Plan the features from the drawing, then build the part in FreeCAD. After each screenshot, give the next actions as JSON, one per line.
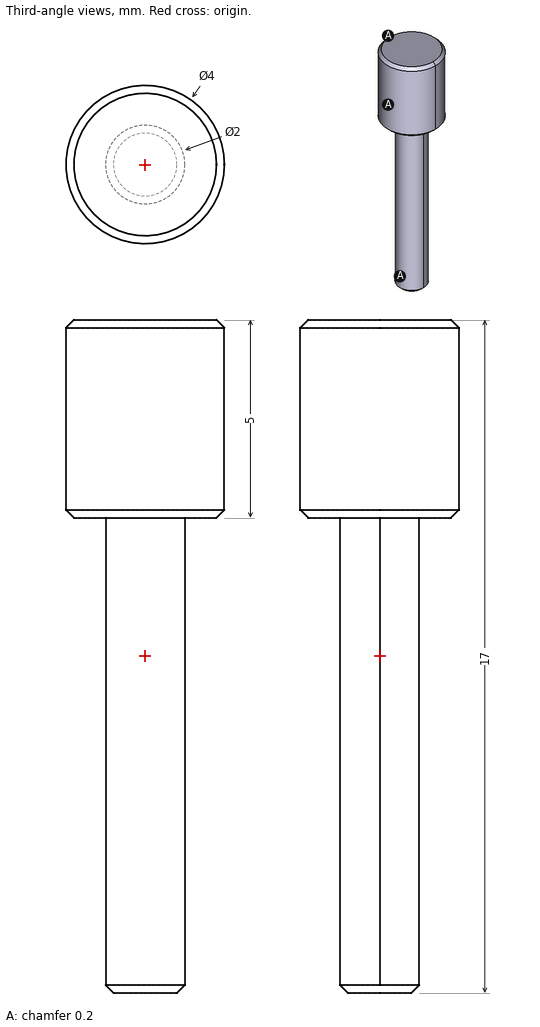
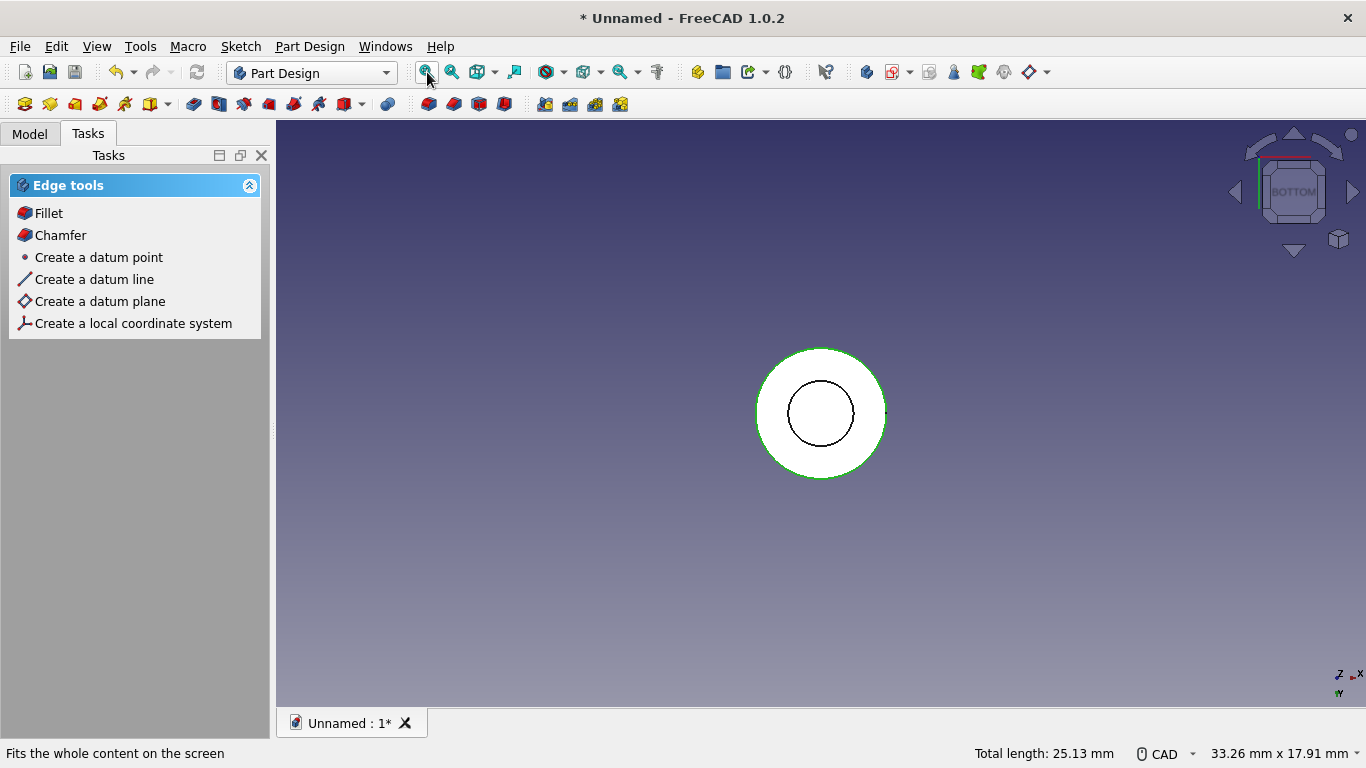
{"action": "left_click", "coordinate": [788, 412], "text": "ctrl"}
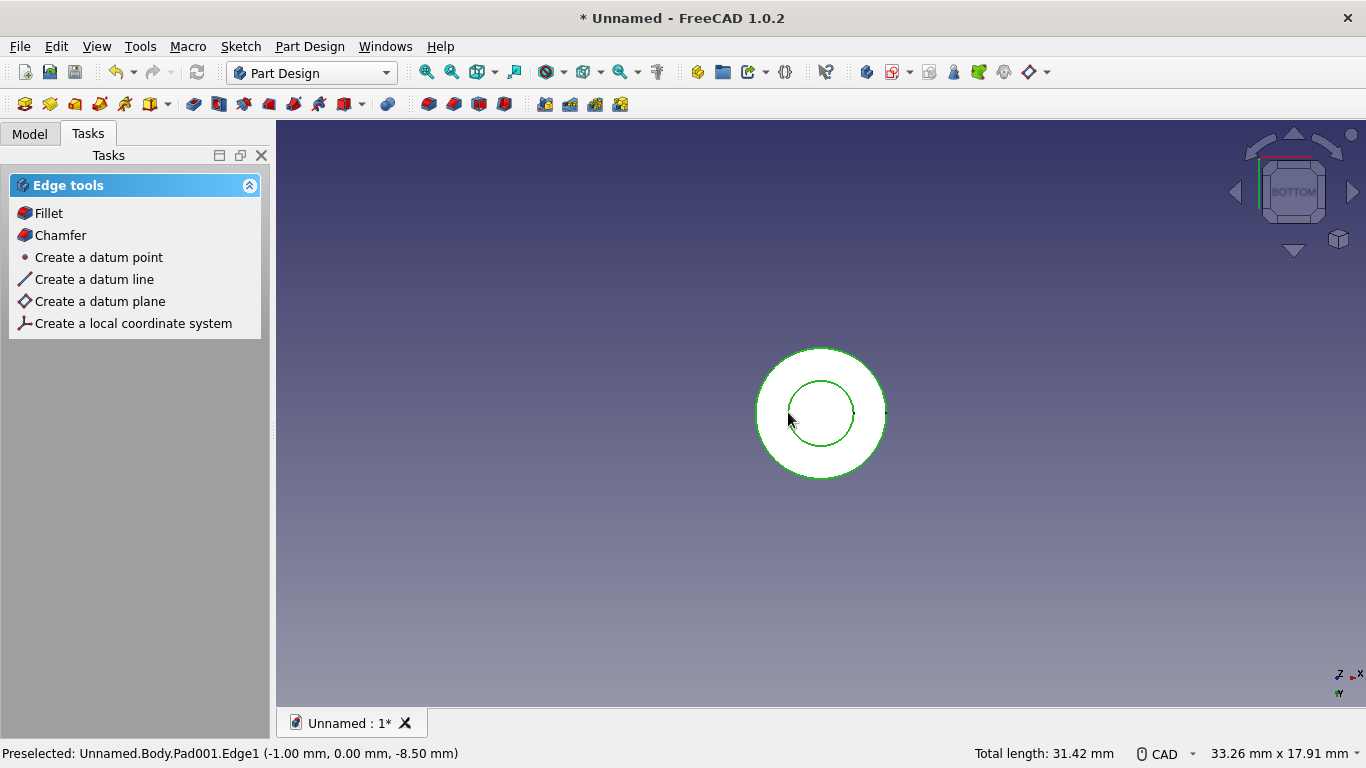
{"action": "left_click", "coordinate": [454, 104]}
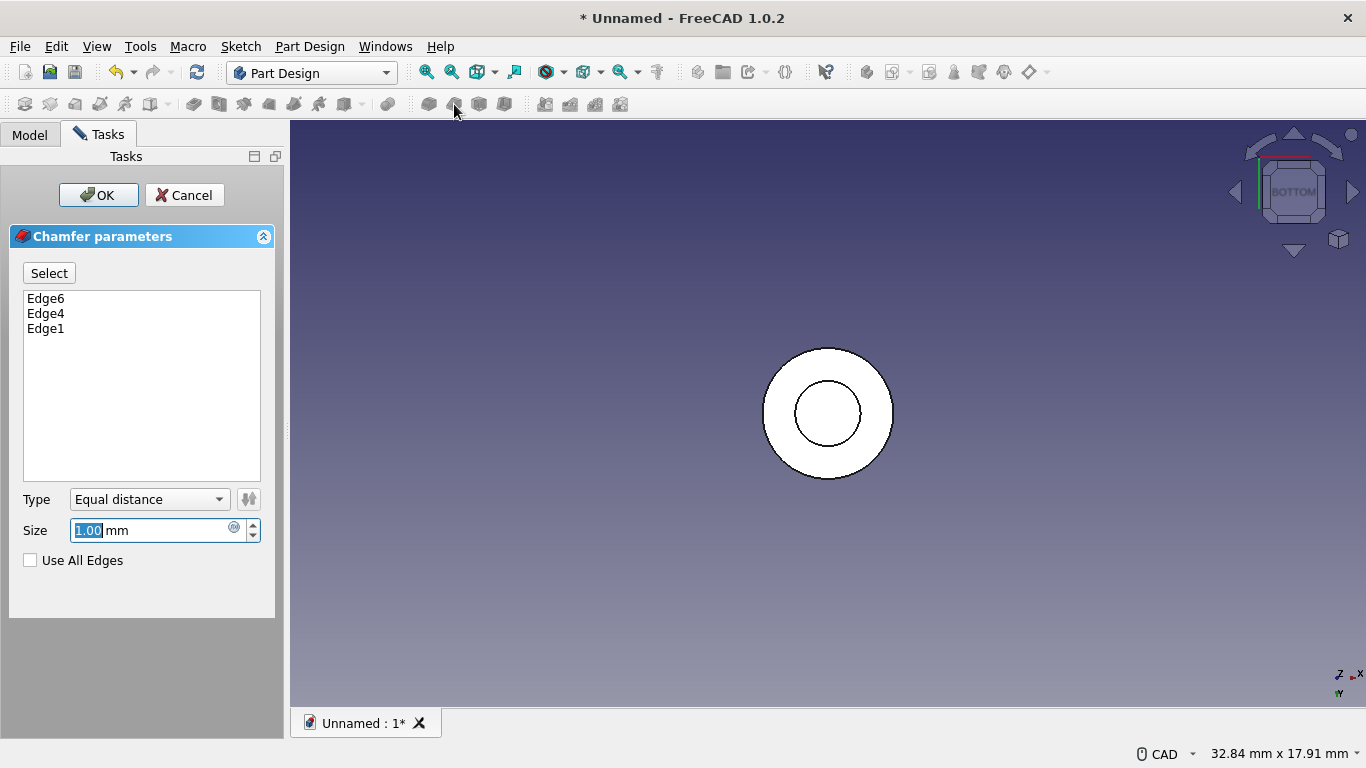
{"action": "type", "text": "0.2"}
{"action": "key", "text": "Tab"}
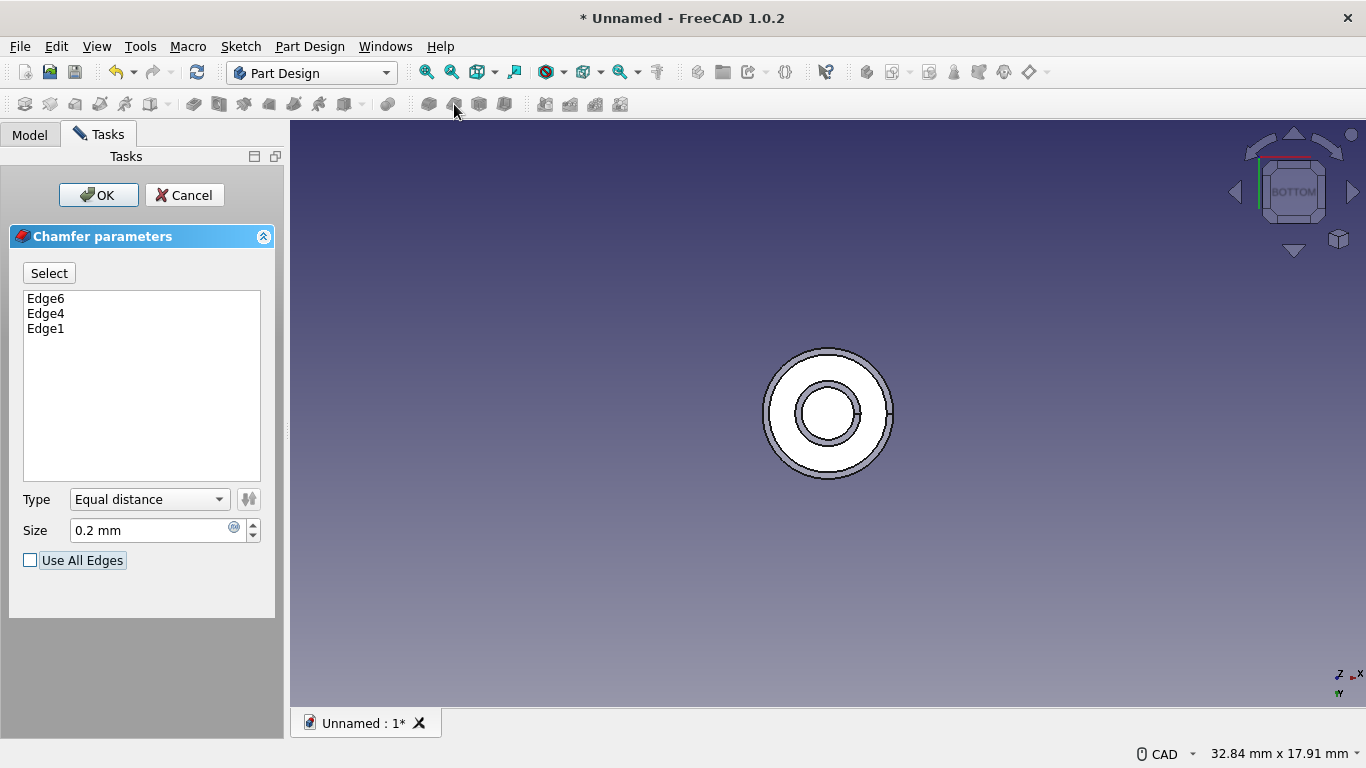
{"action": "left_click", "coordinate": [99, 195]}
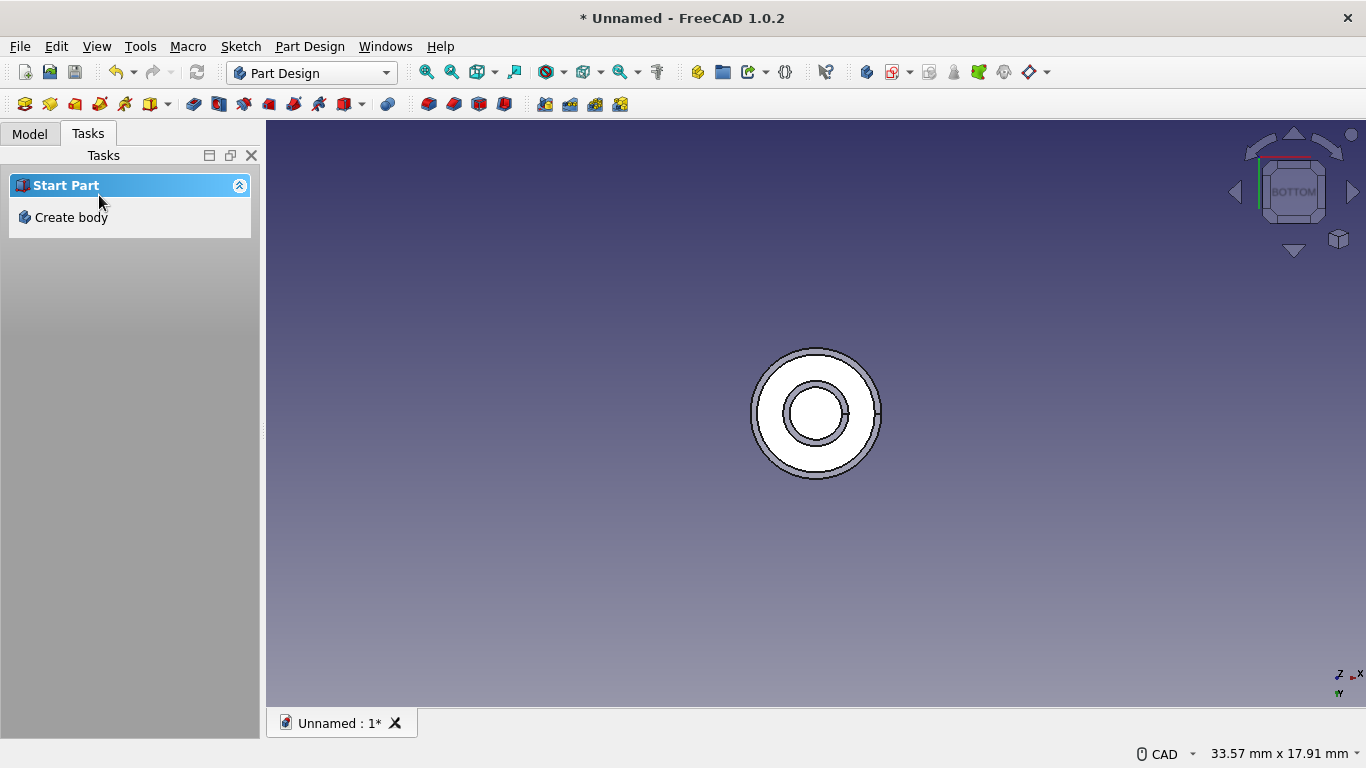
{"action": "key", "text": "0"}